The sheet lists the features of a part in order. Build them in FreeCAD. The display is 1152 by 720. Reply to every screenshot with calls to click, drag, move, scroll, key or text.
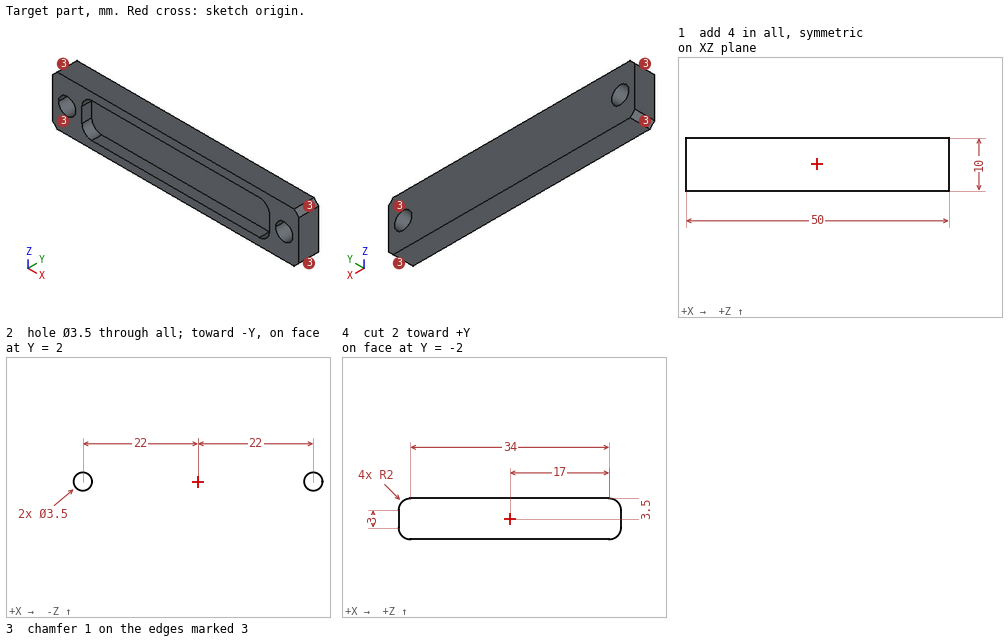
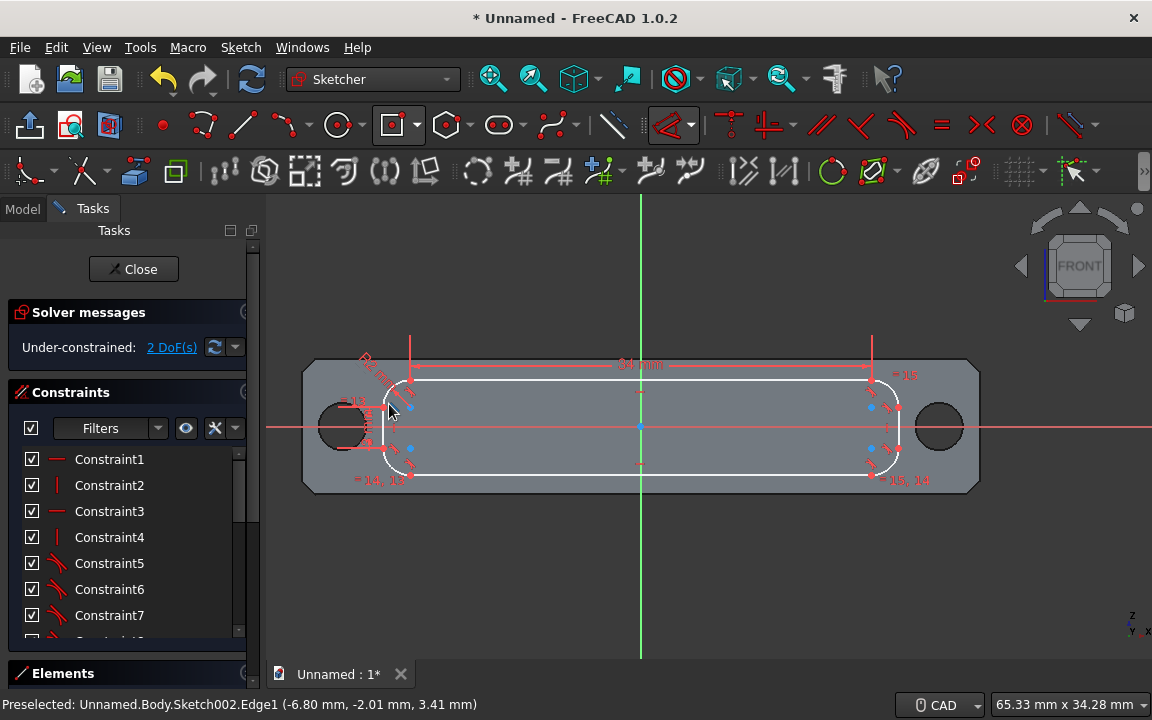
click(872, 380)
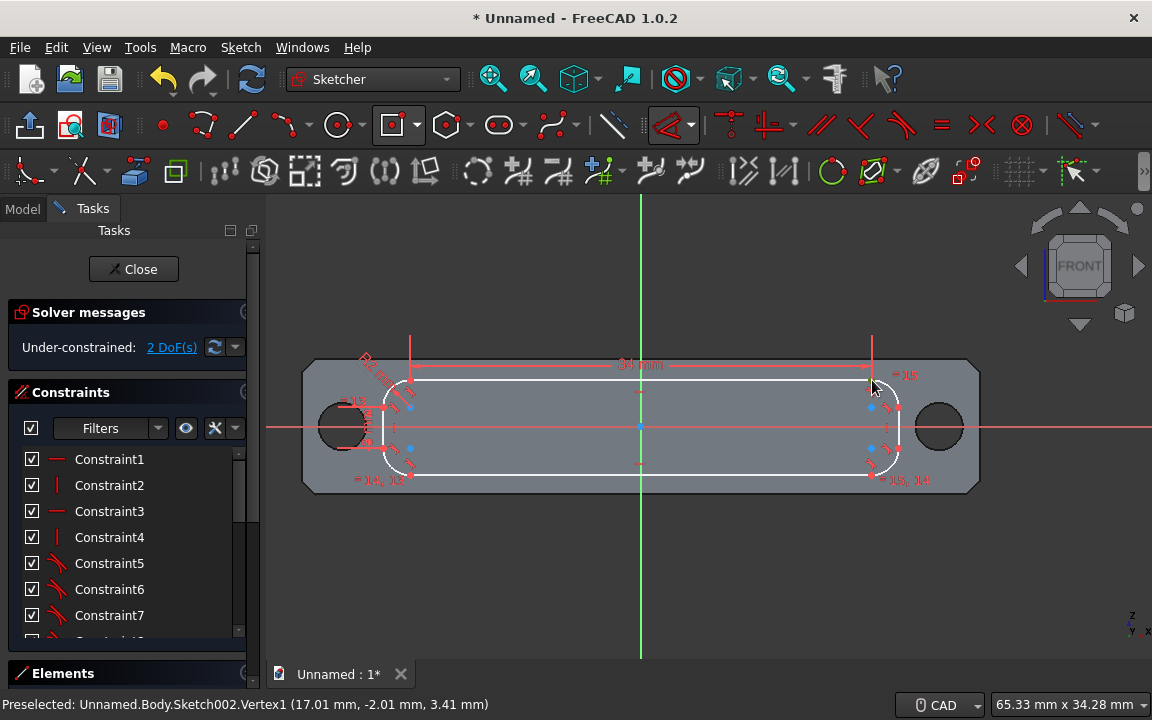
click(694, 126)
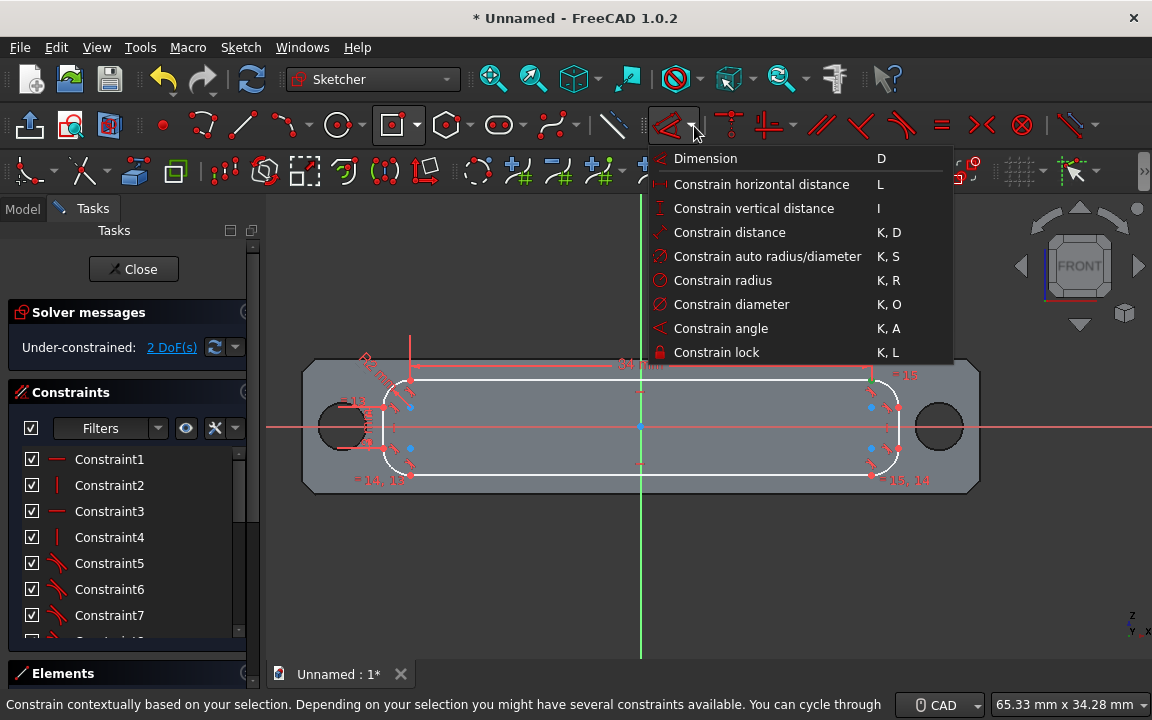
click(801, 184)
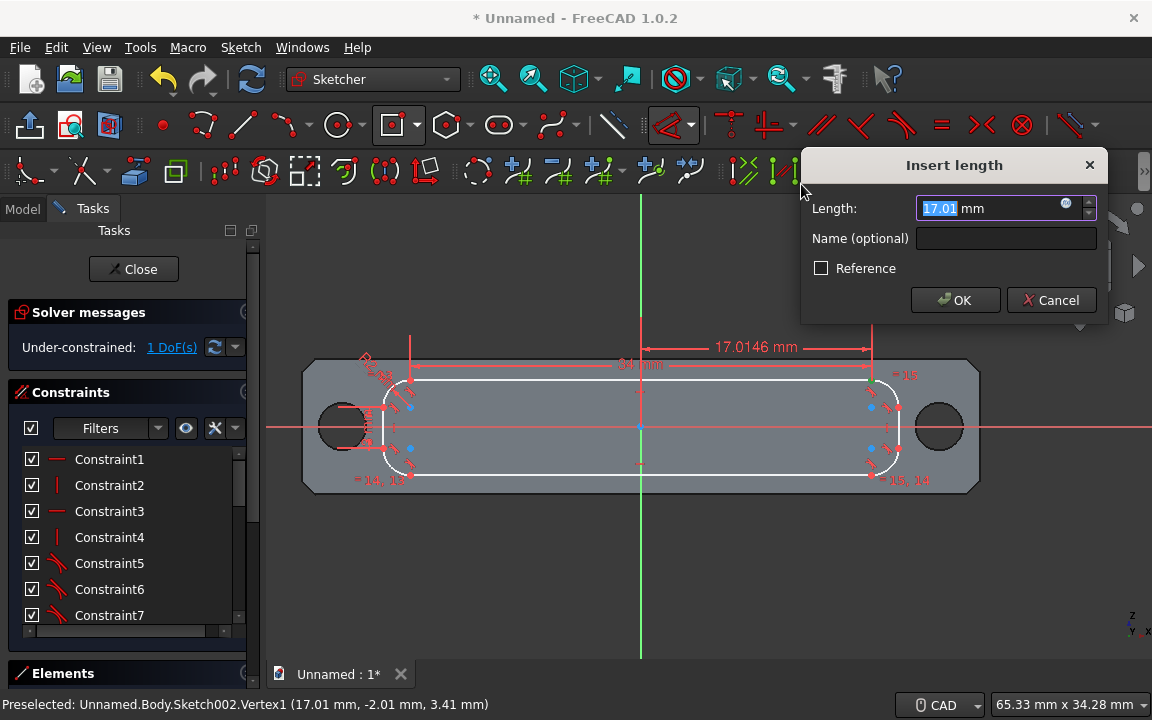
text(17)
key(Return)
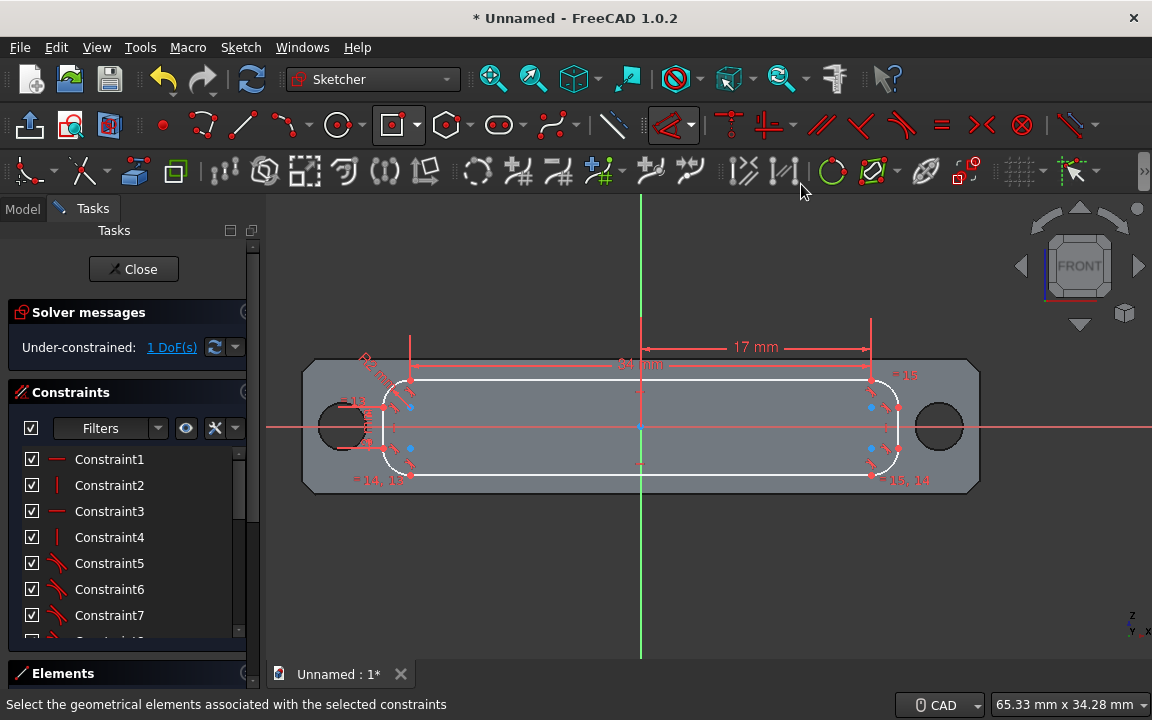
click(871, 380)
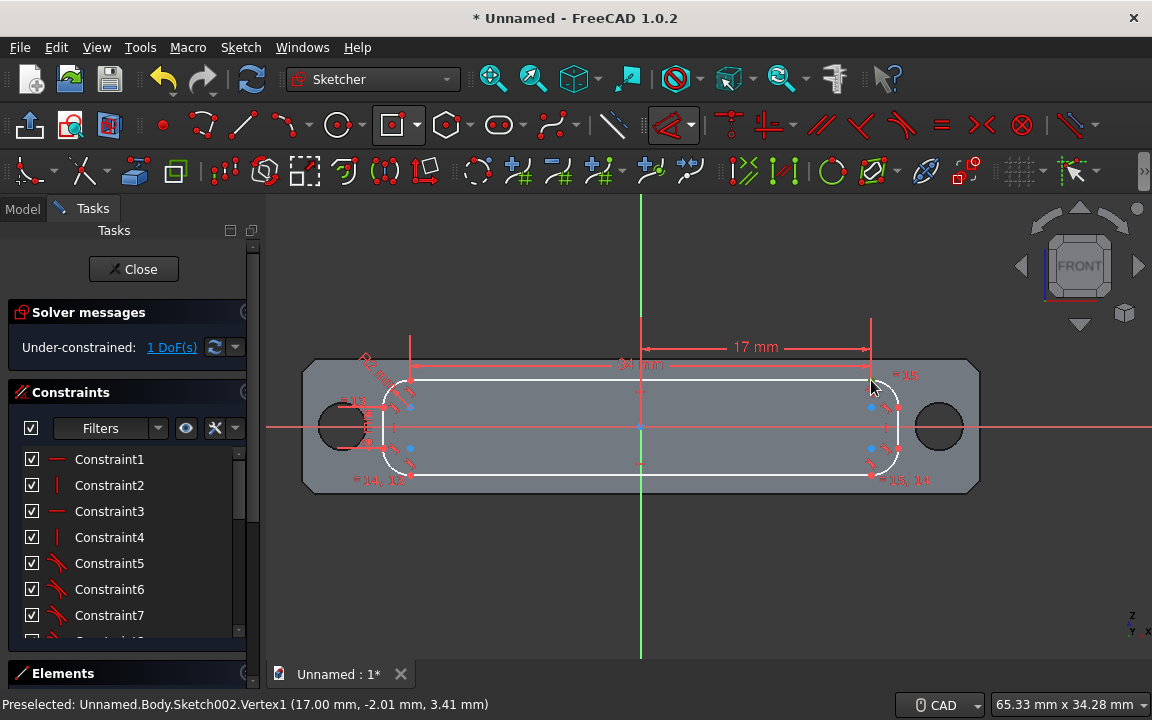
click(694, 126)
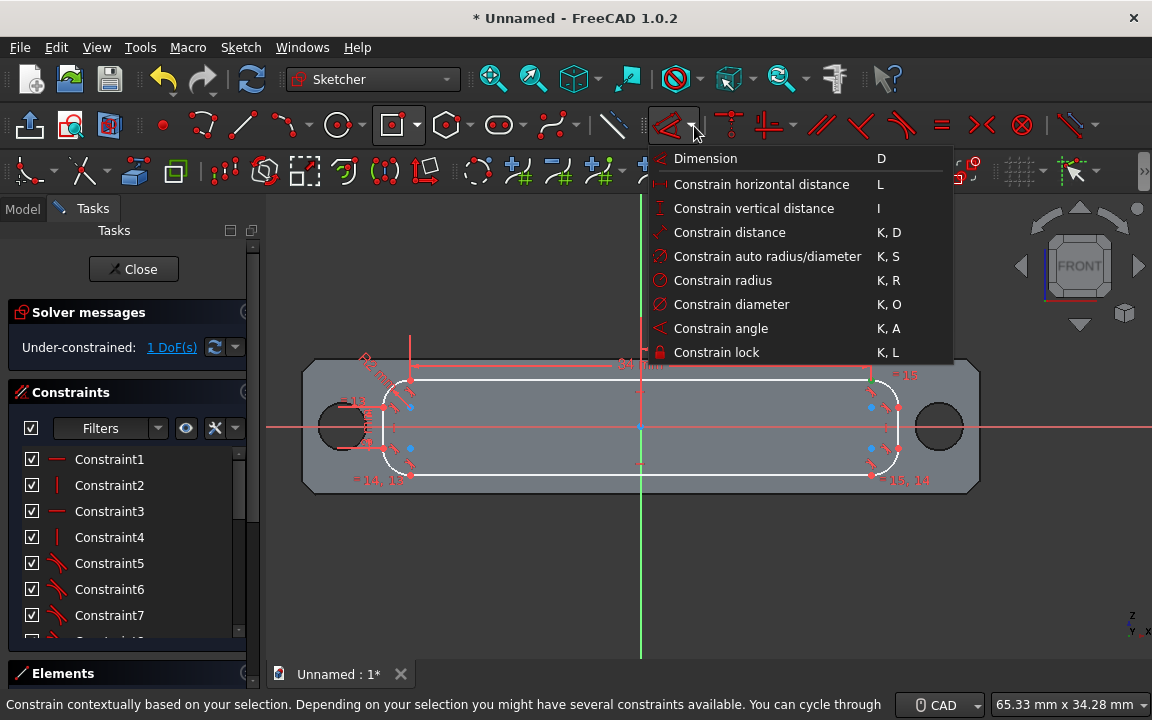
click(801, 208)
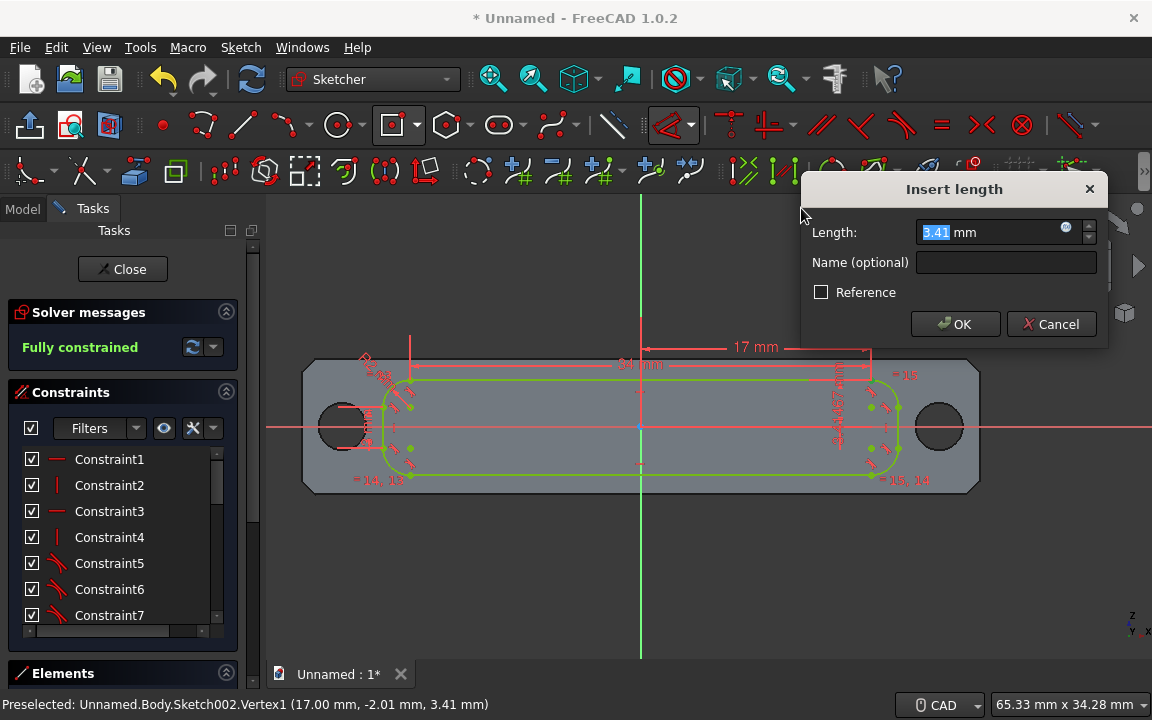
text(3.5)
key(Return)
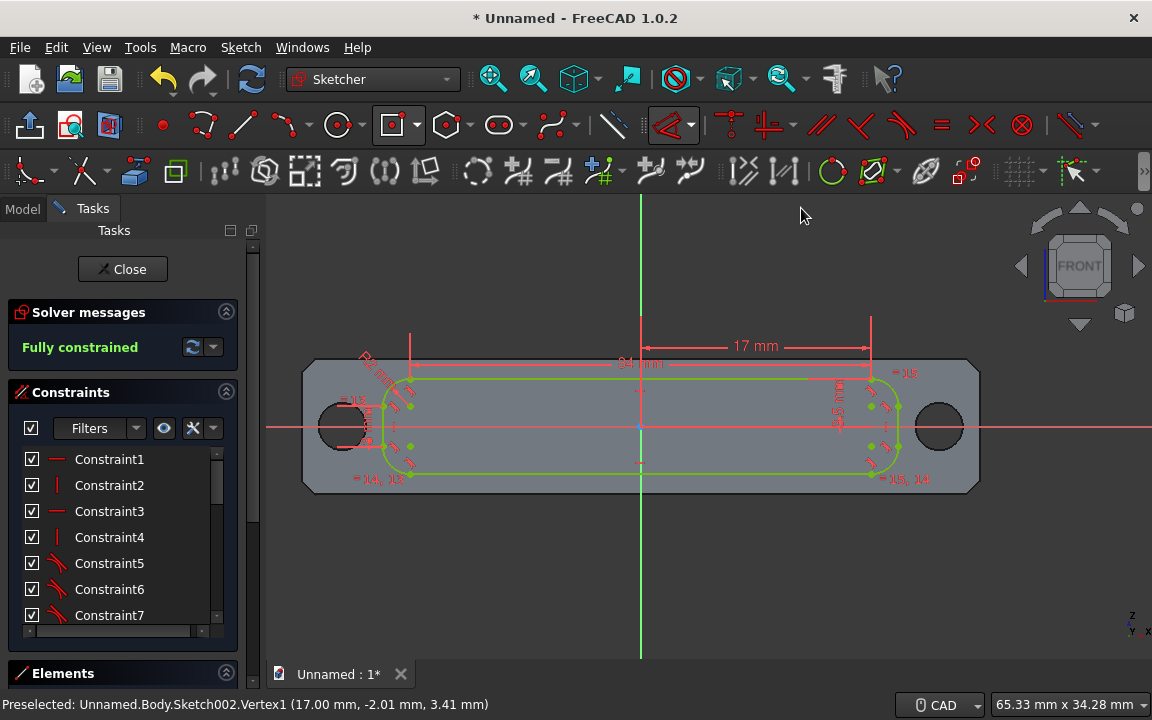
click(123, 269)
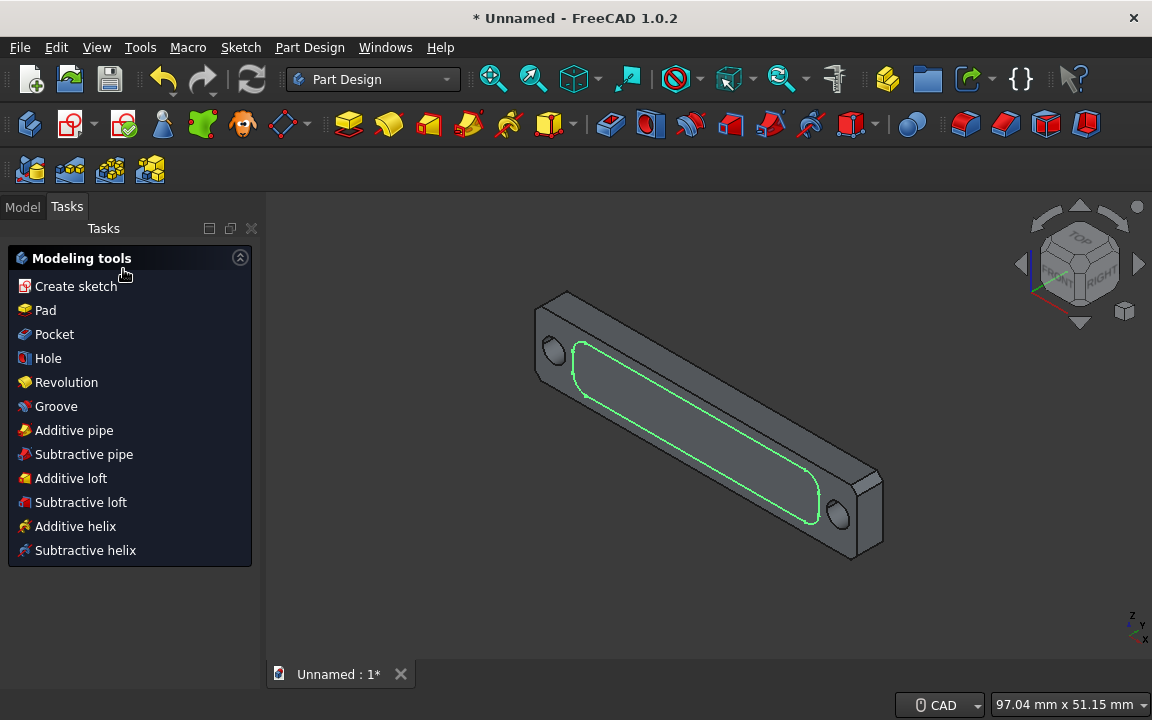
click(612, 124)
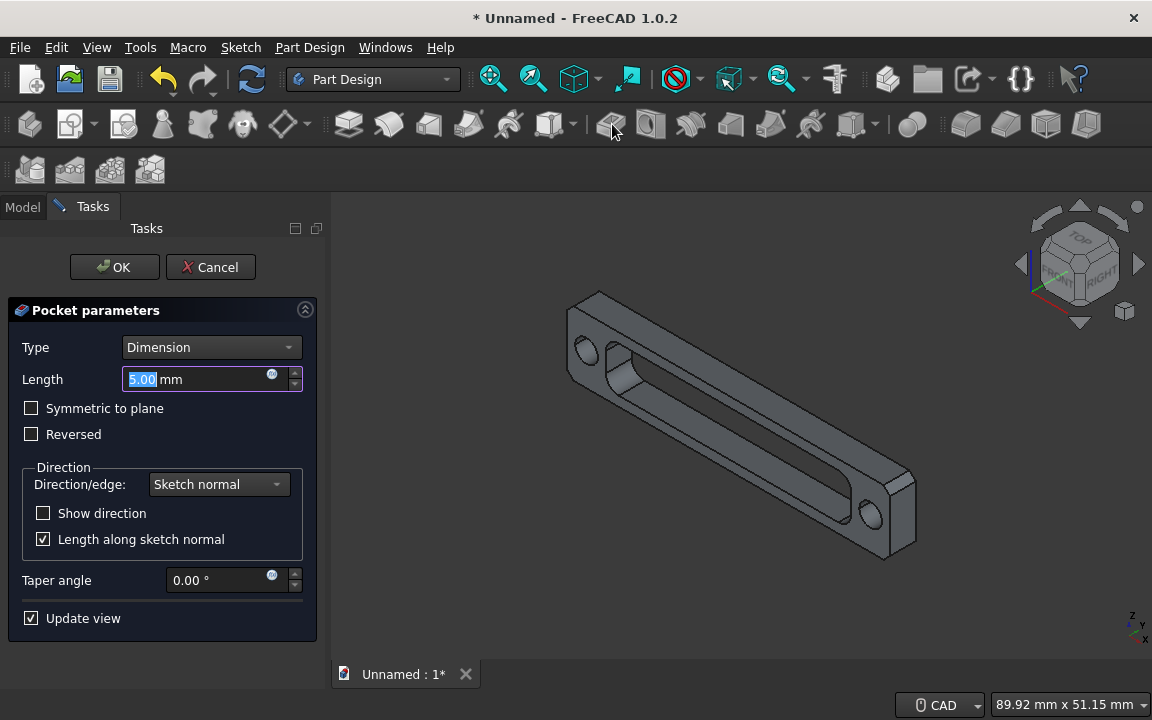
text(2)
key(Tab)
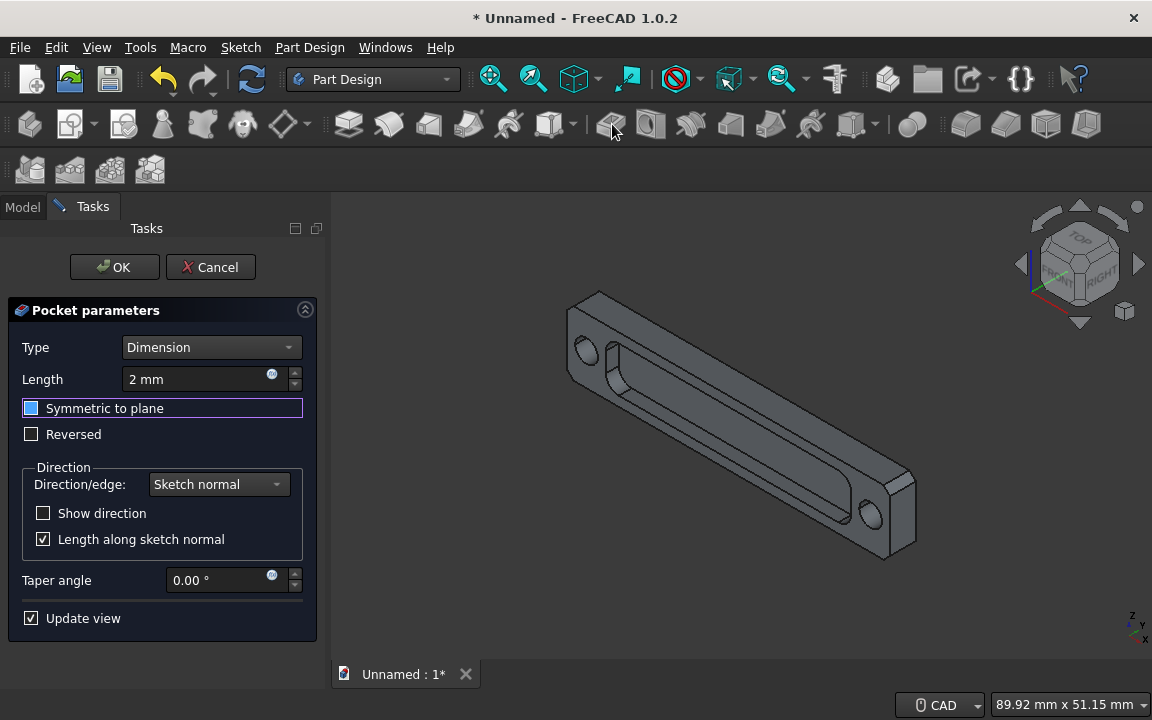
click(115, 267)